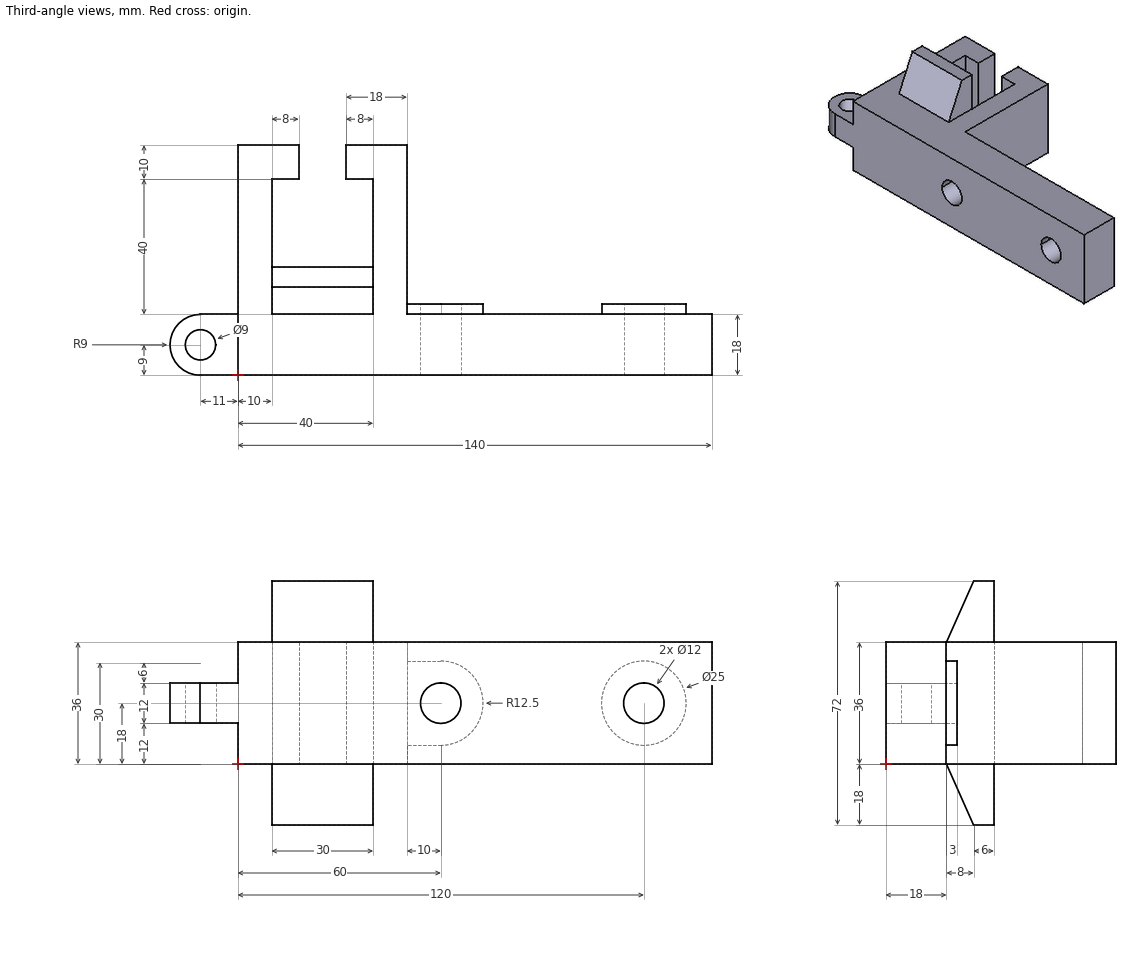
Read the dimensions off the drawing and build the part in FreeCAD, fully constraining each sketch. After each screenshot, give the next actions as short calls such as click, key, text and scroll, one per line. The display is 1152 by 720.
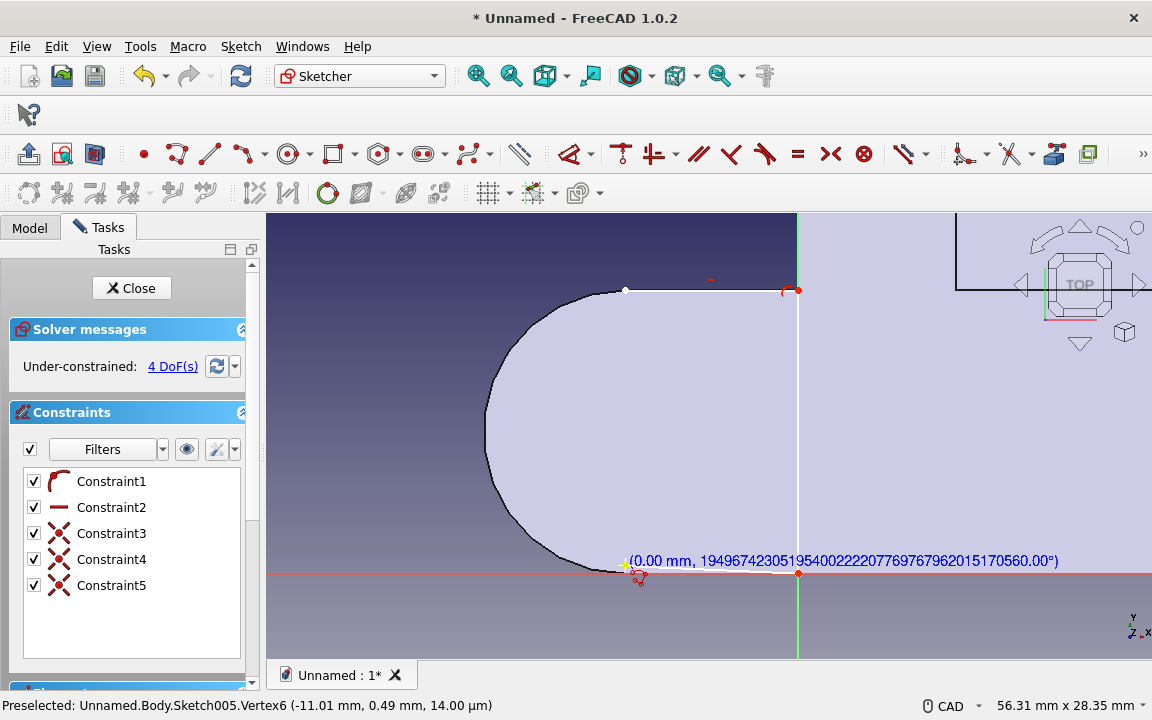
key(g)
key(3)
key(a)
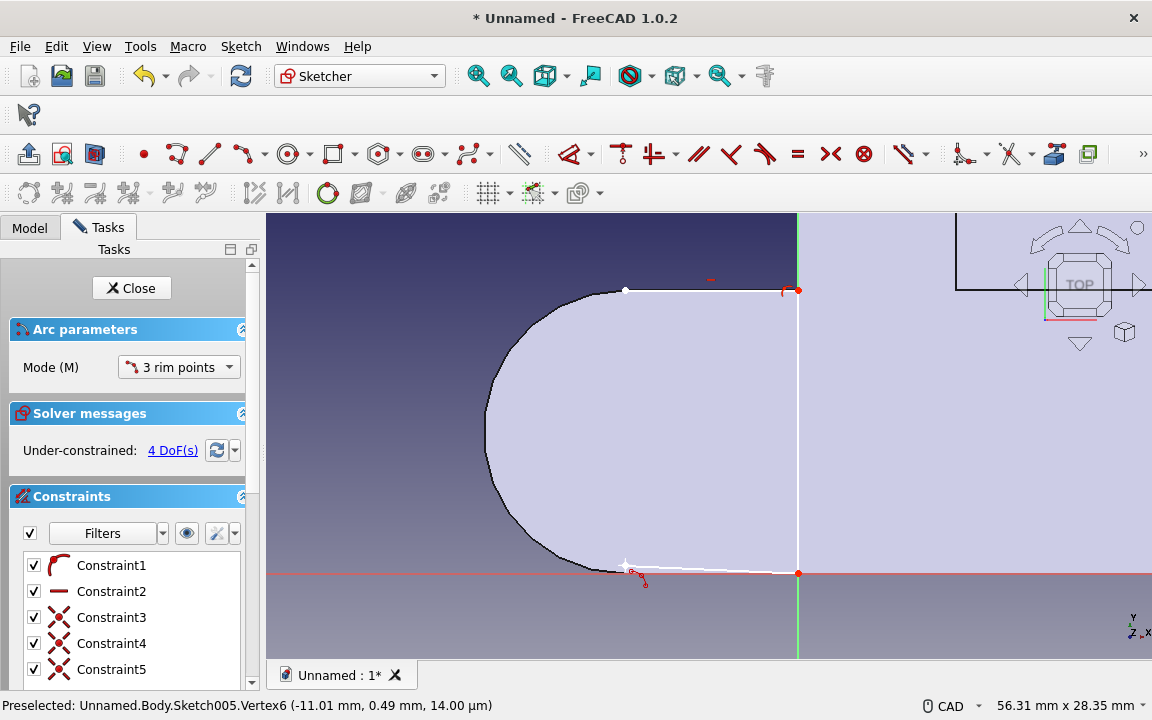
click(625, 566)
click(625, 291)
click(483, 432)
key(Escape)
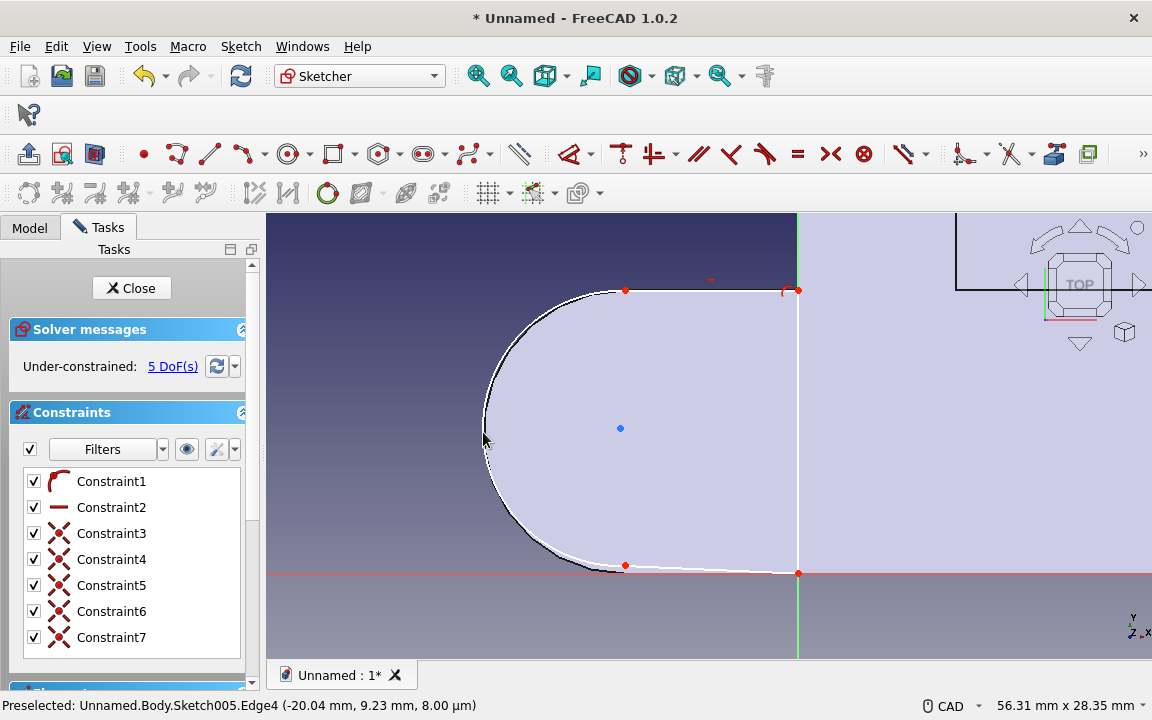
click(677, 291)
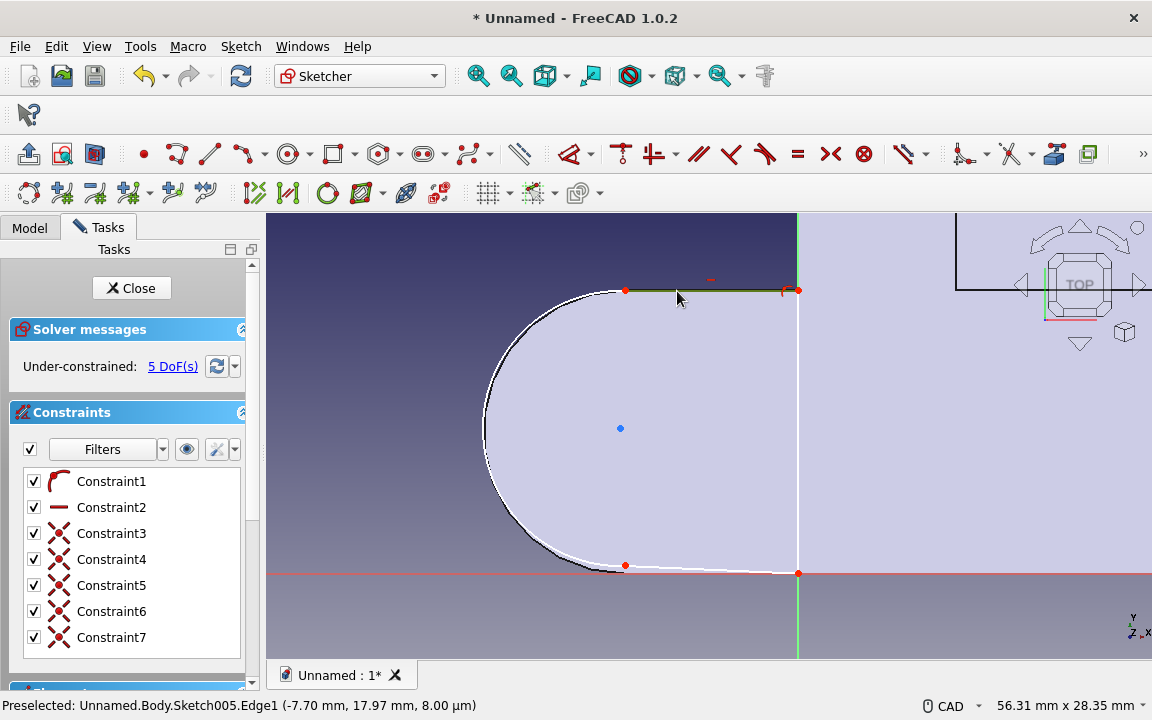
click(510, 346)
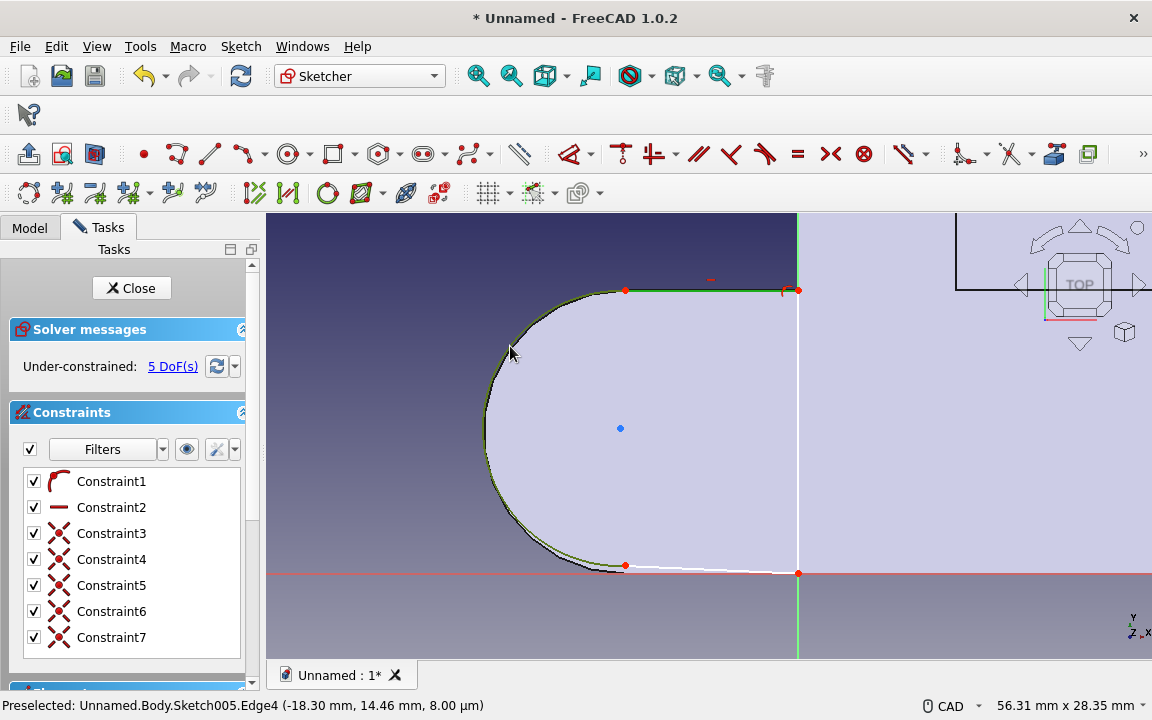
click(765, 154)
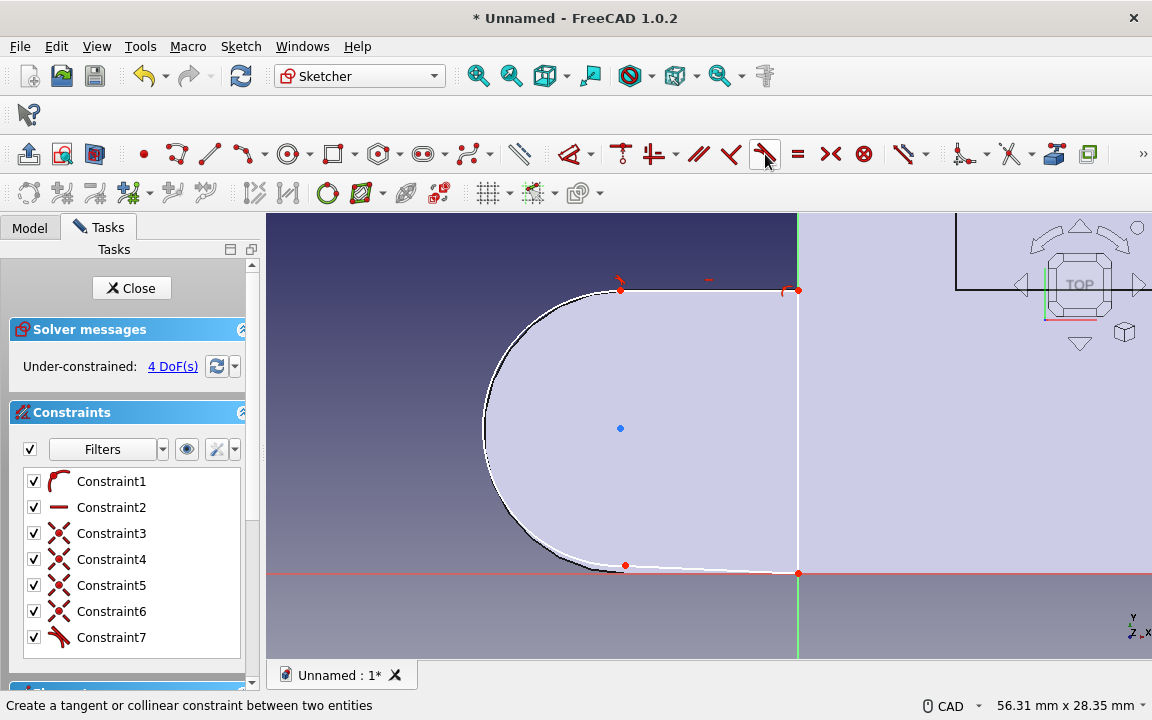
click(746, 571)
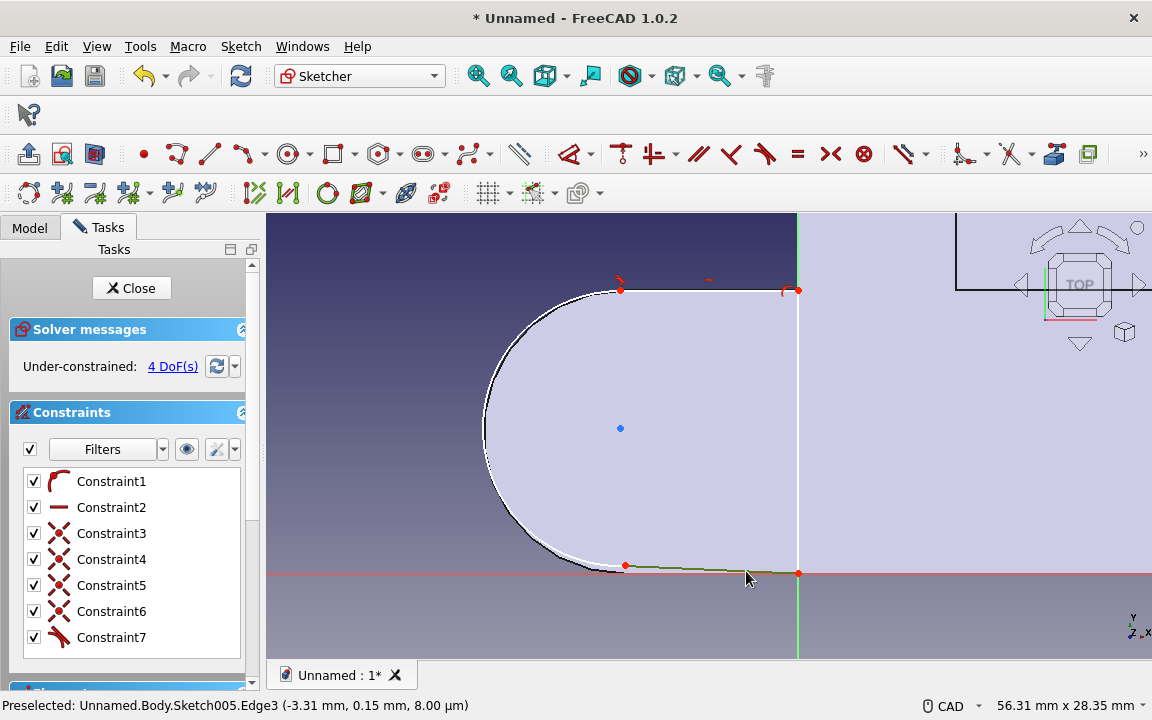
click(508, 349)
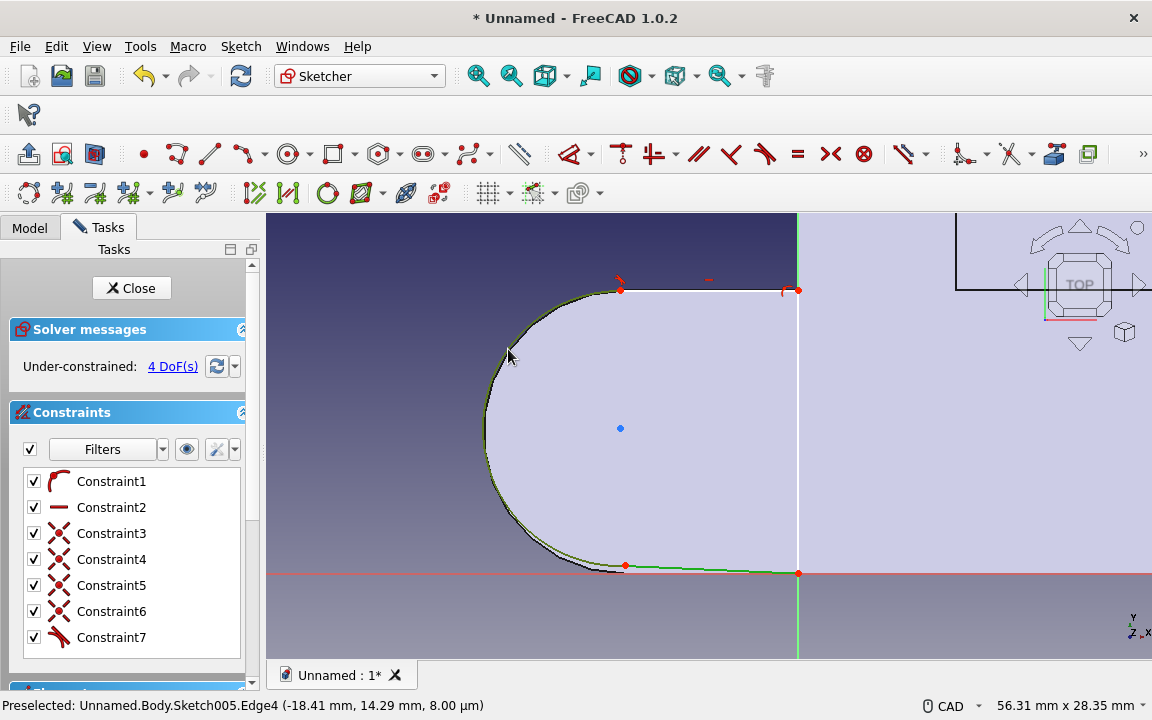
key(t)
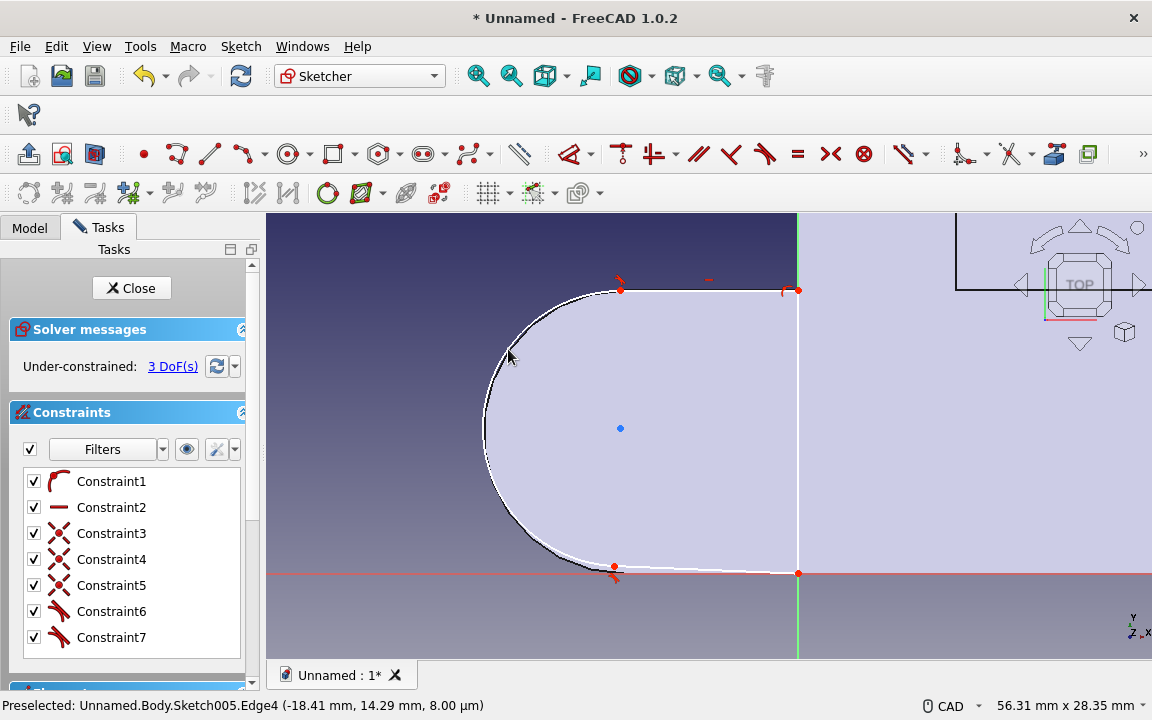
click(743, 571)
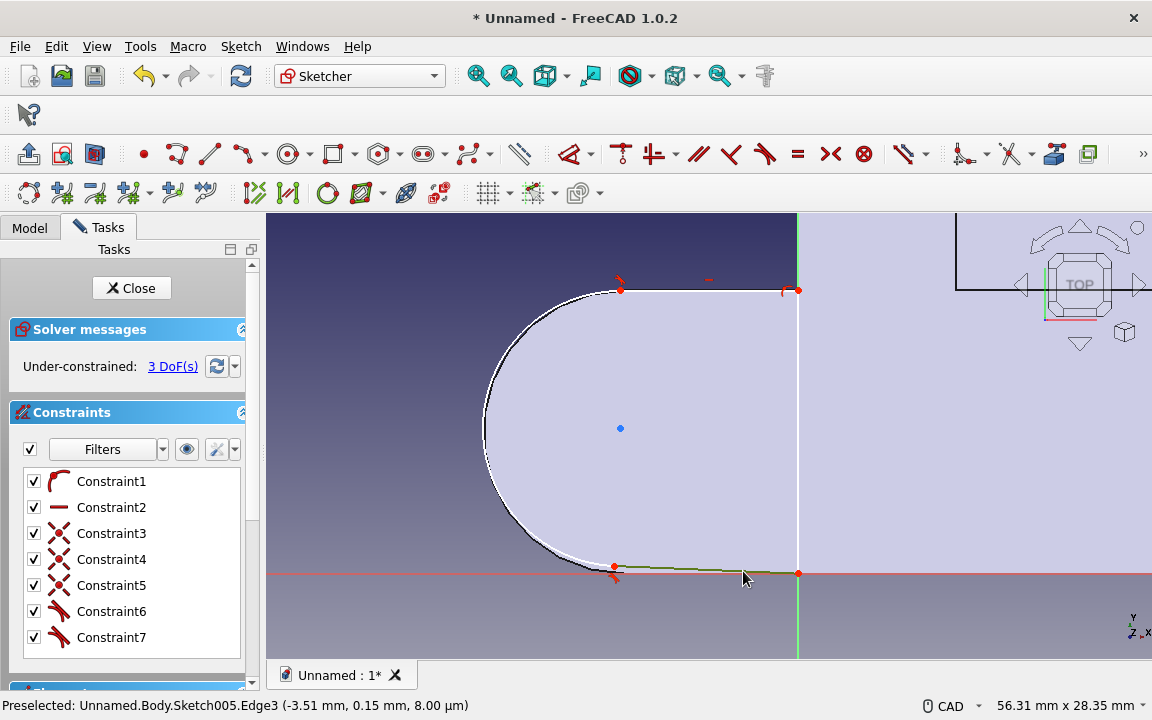
key(h)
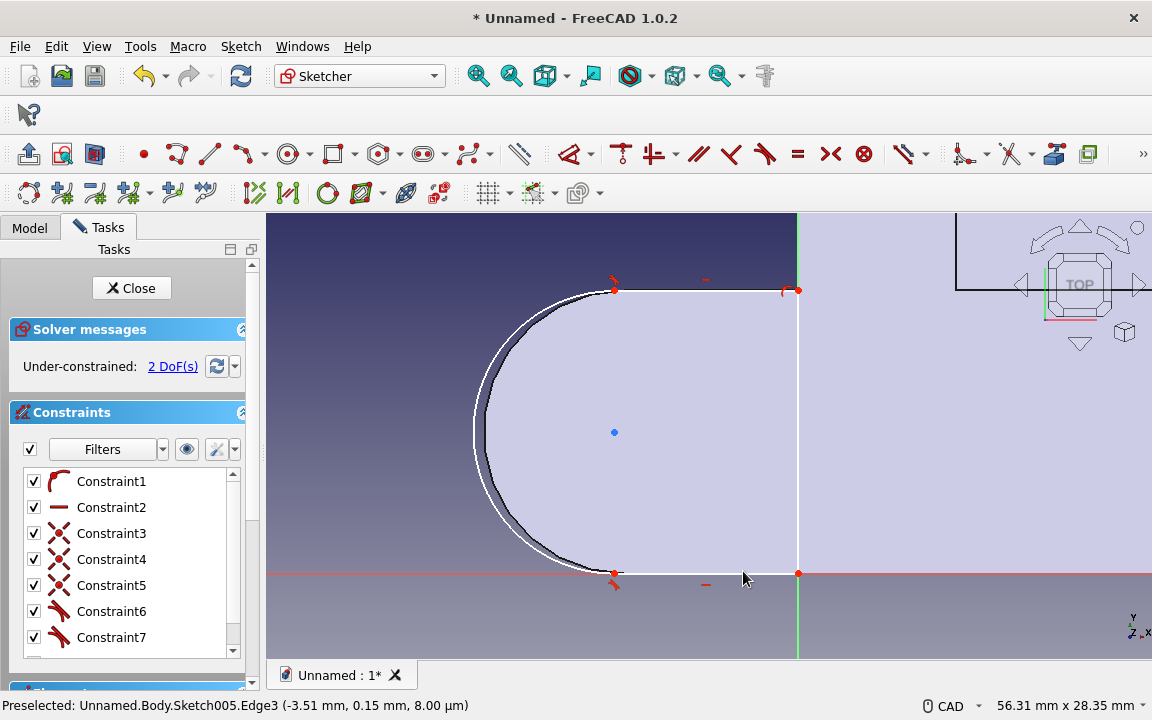
click(568, 154)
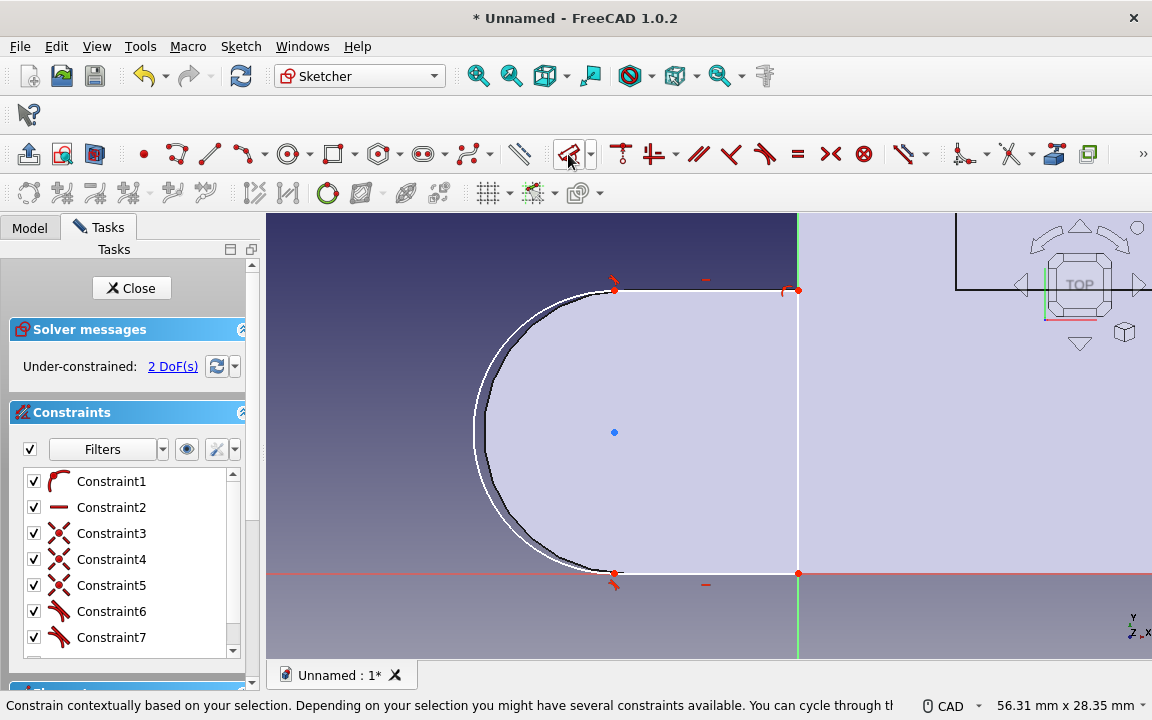
click(501, 349)
click(475, 330)